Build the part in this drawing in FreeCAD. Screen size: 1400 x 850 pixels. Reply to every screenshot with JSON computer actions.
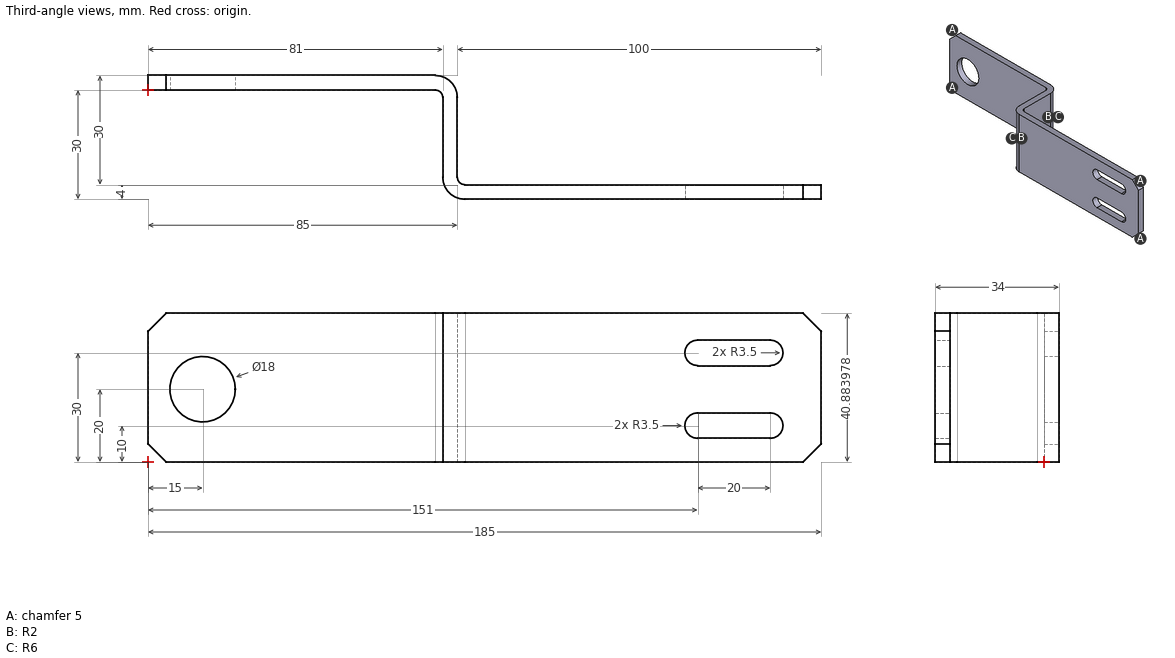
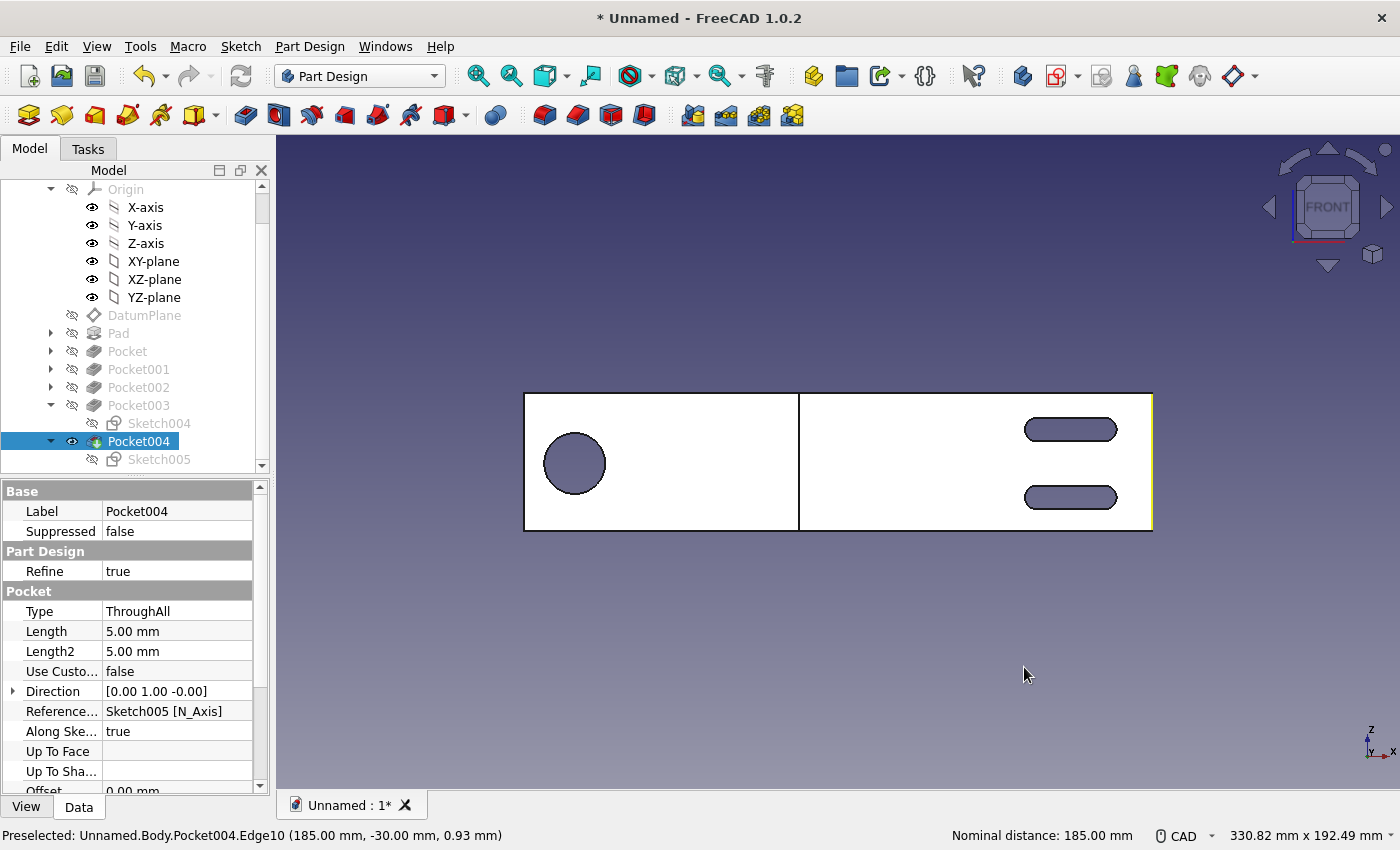
{"action": "scroll", "coordinate": [1152, 530], "scroll_direction": "up", "scroll_amount": 6}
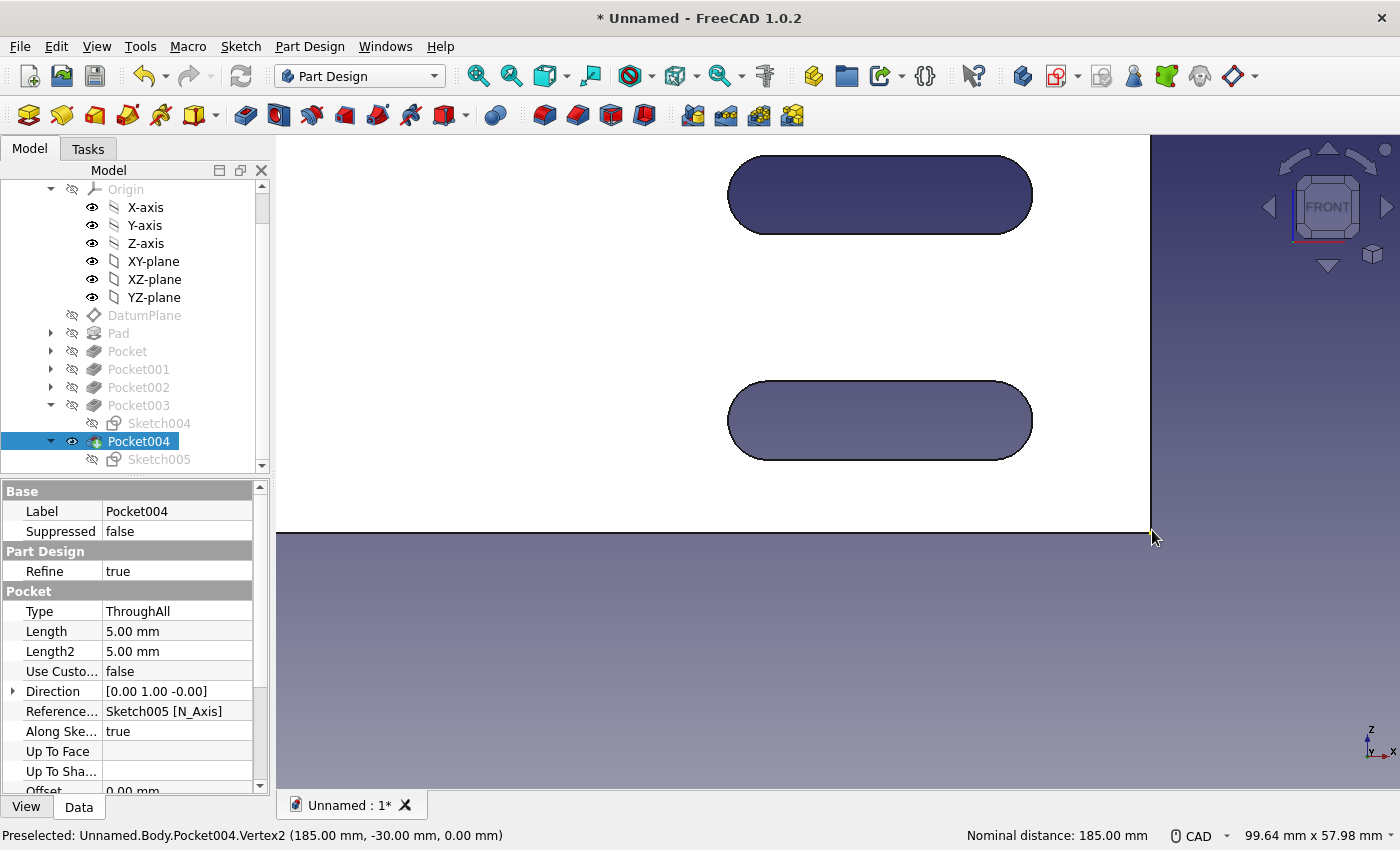
{"action": "key", "text": "v f"}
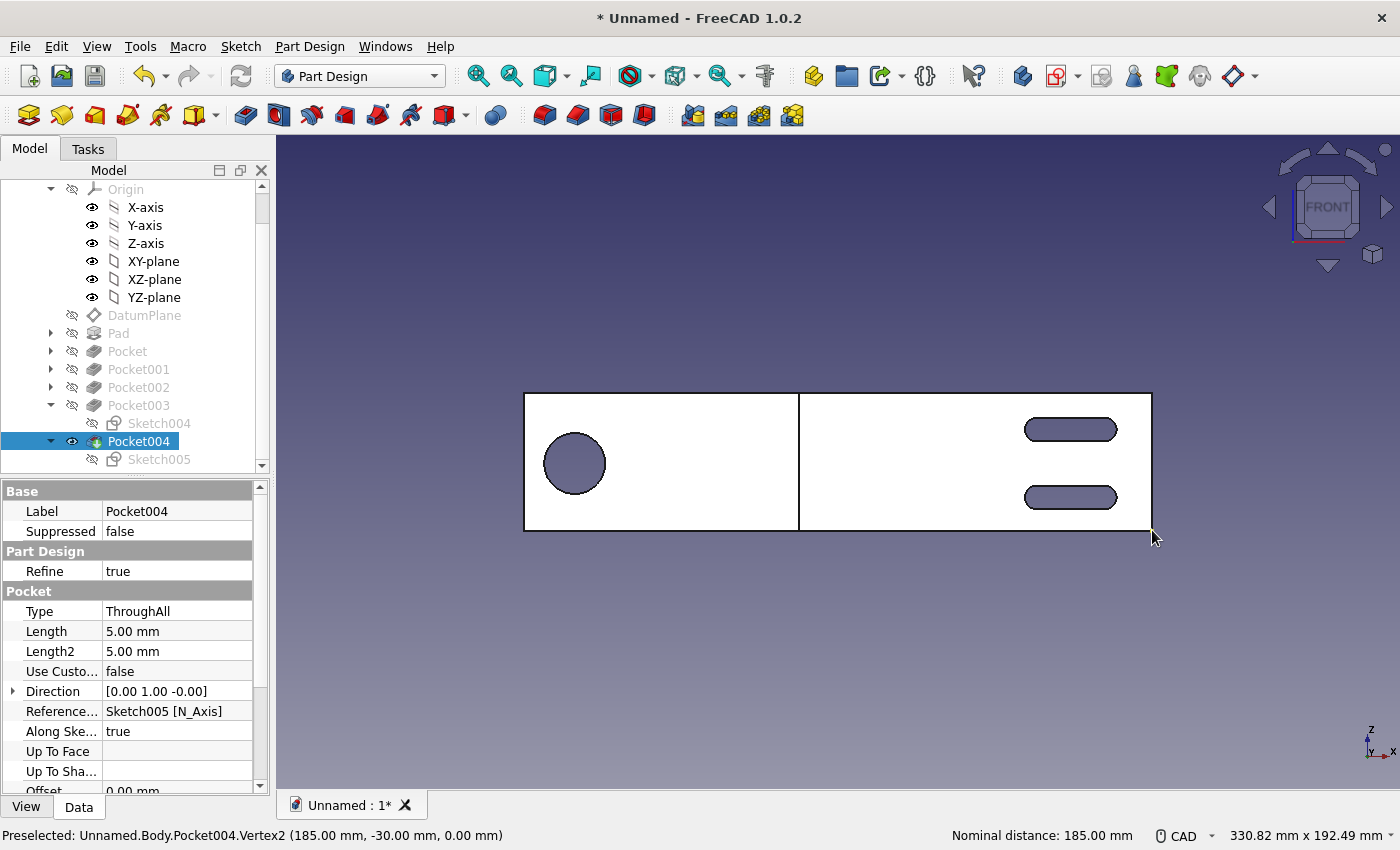
{"action": "key", "text": "3"}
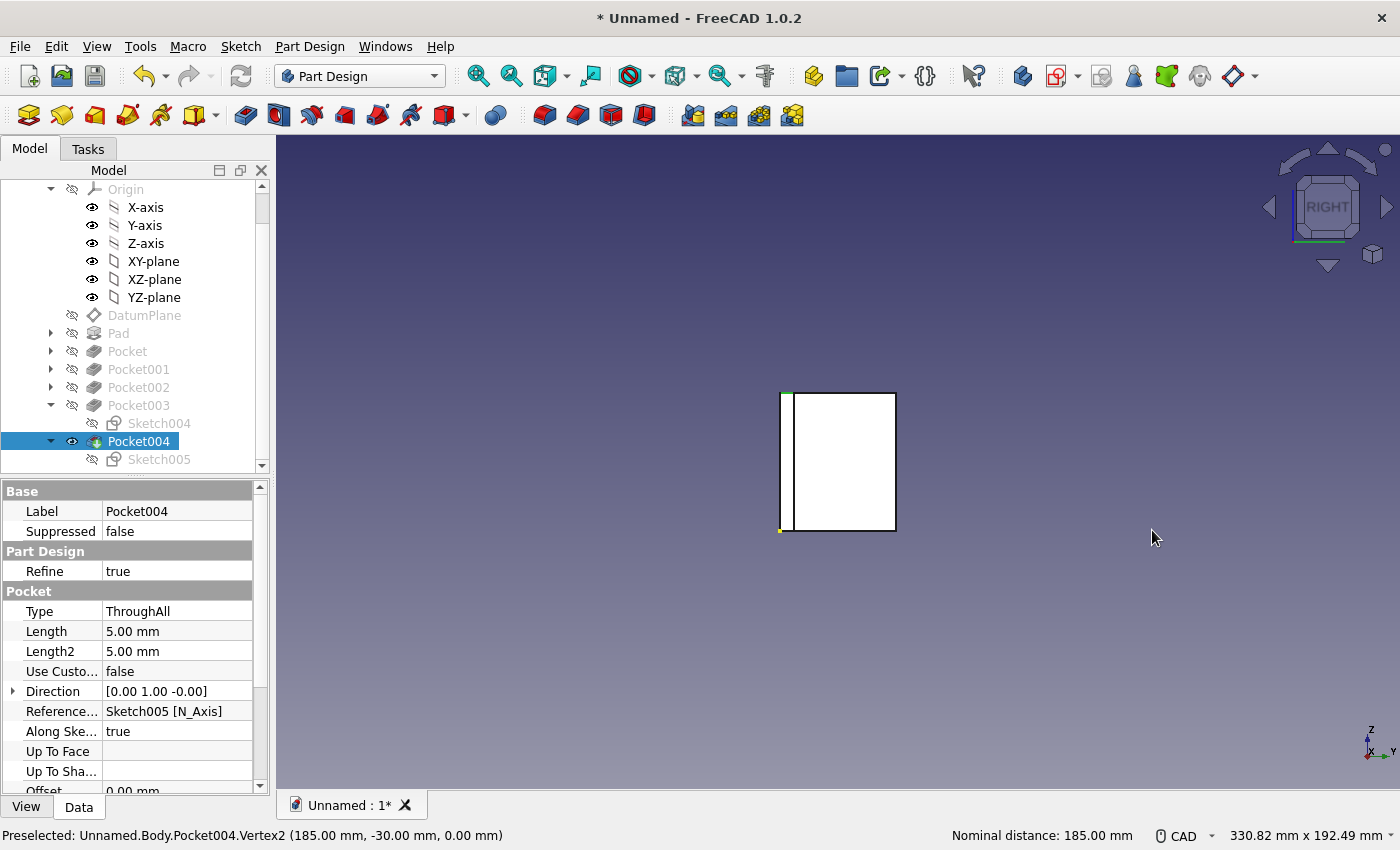
{"action": "left_click", "coordinate": [479, 76]}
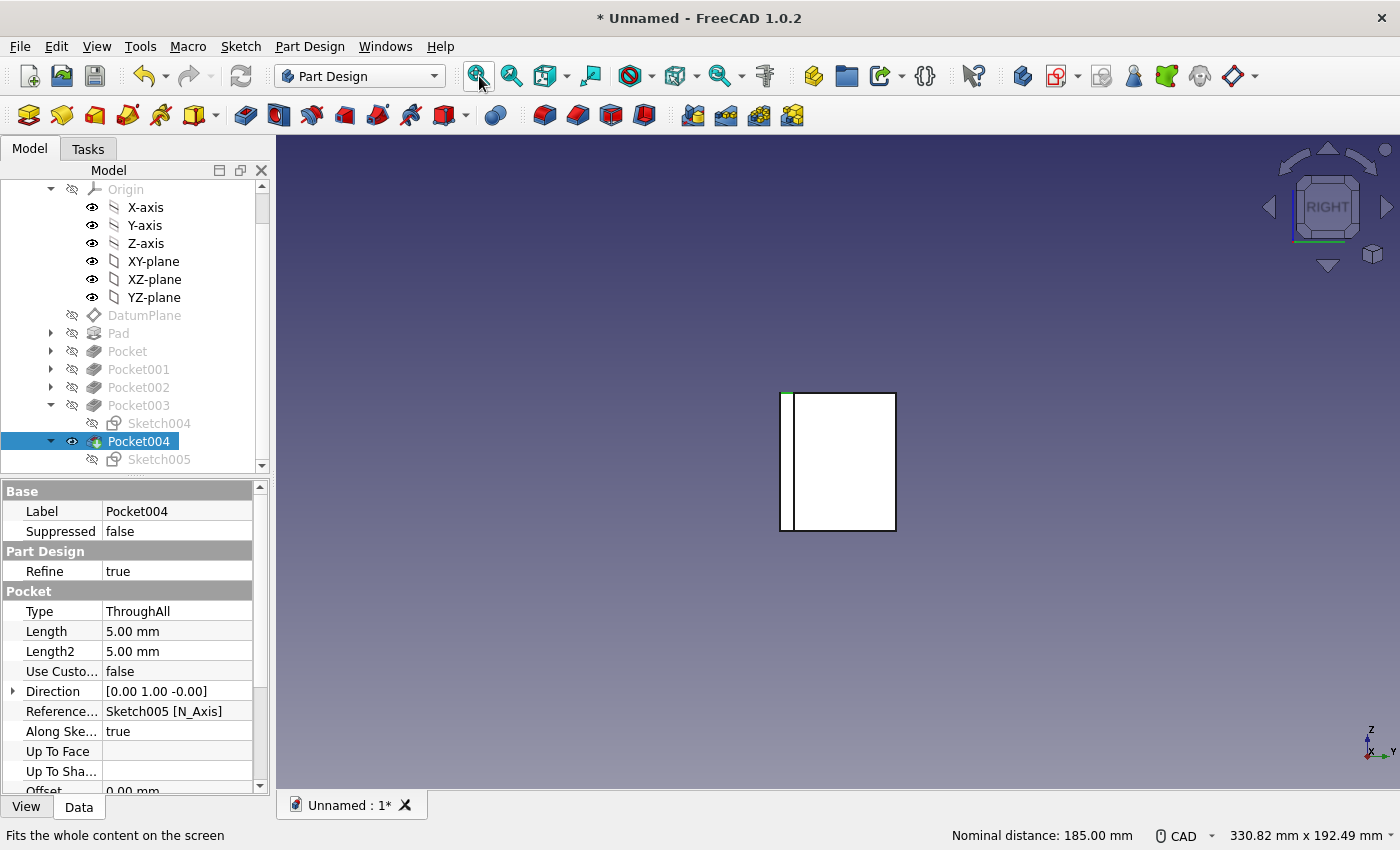
{"action": "left_click", "coordinate": [787, 530], "text": "ctrl"}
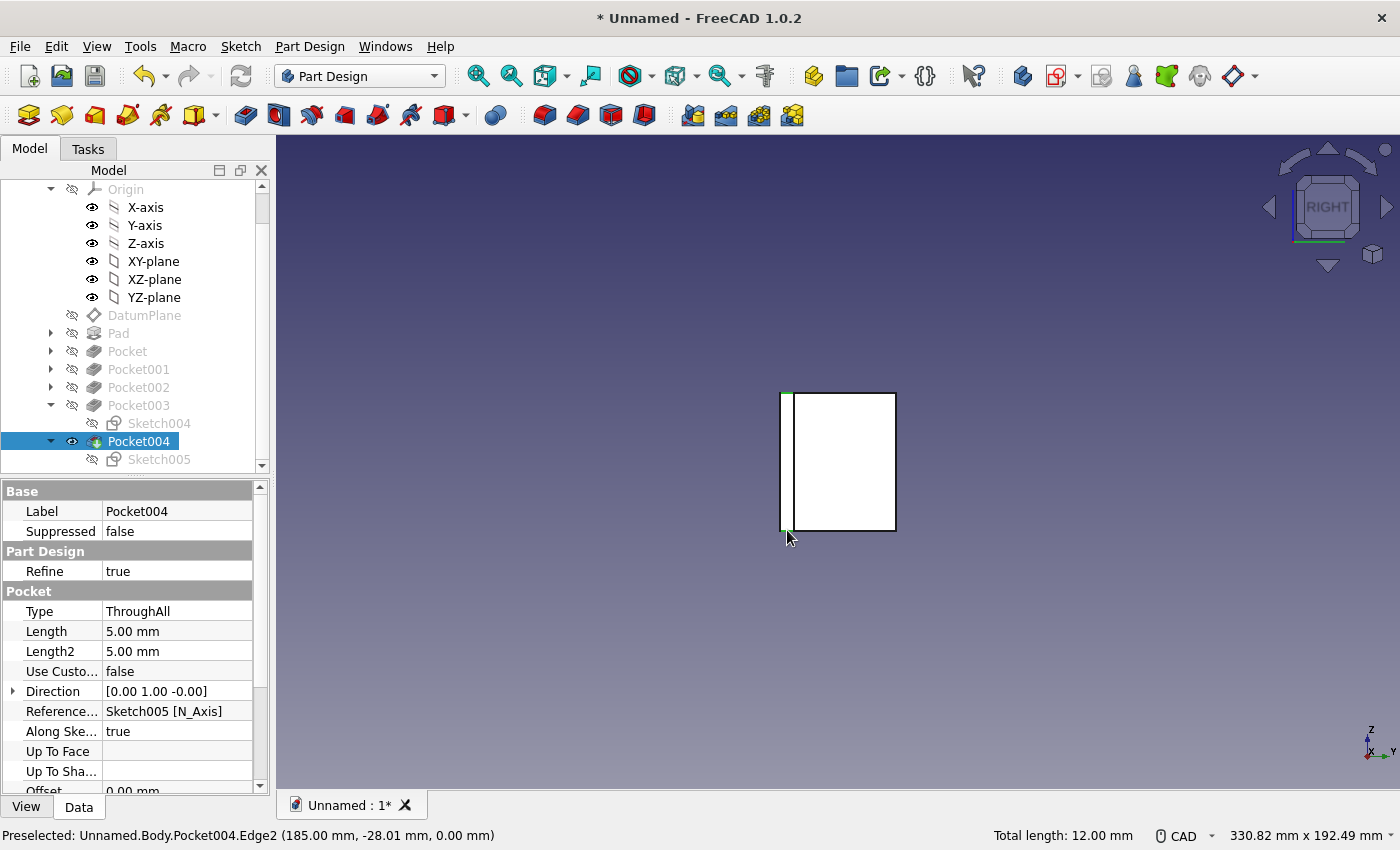
{"action": "scroll", "coordinate": [889, 530], "scroll_direction": "up", "scroll_amount": 6}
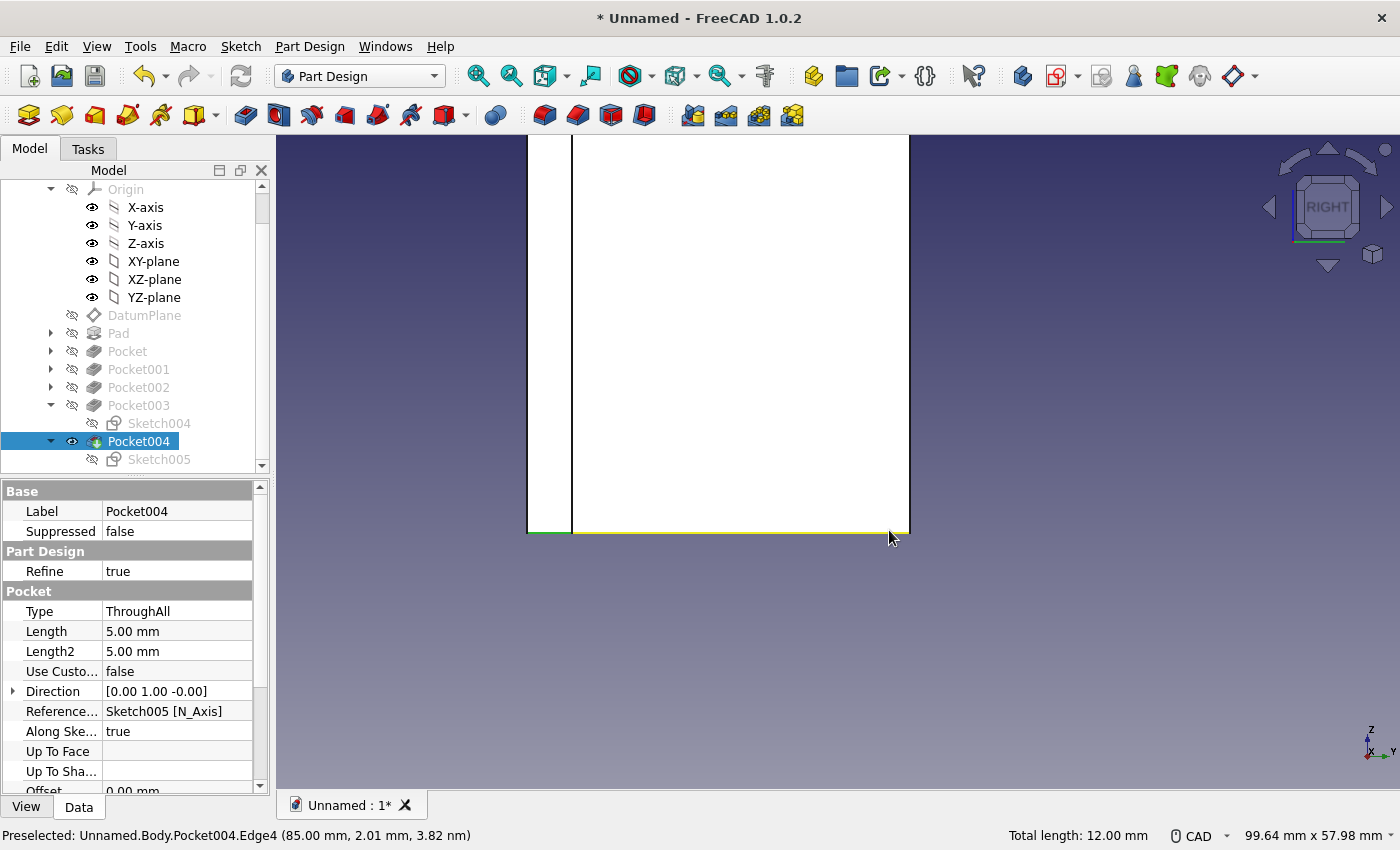
{"action": "key", "text": "v f"}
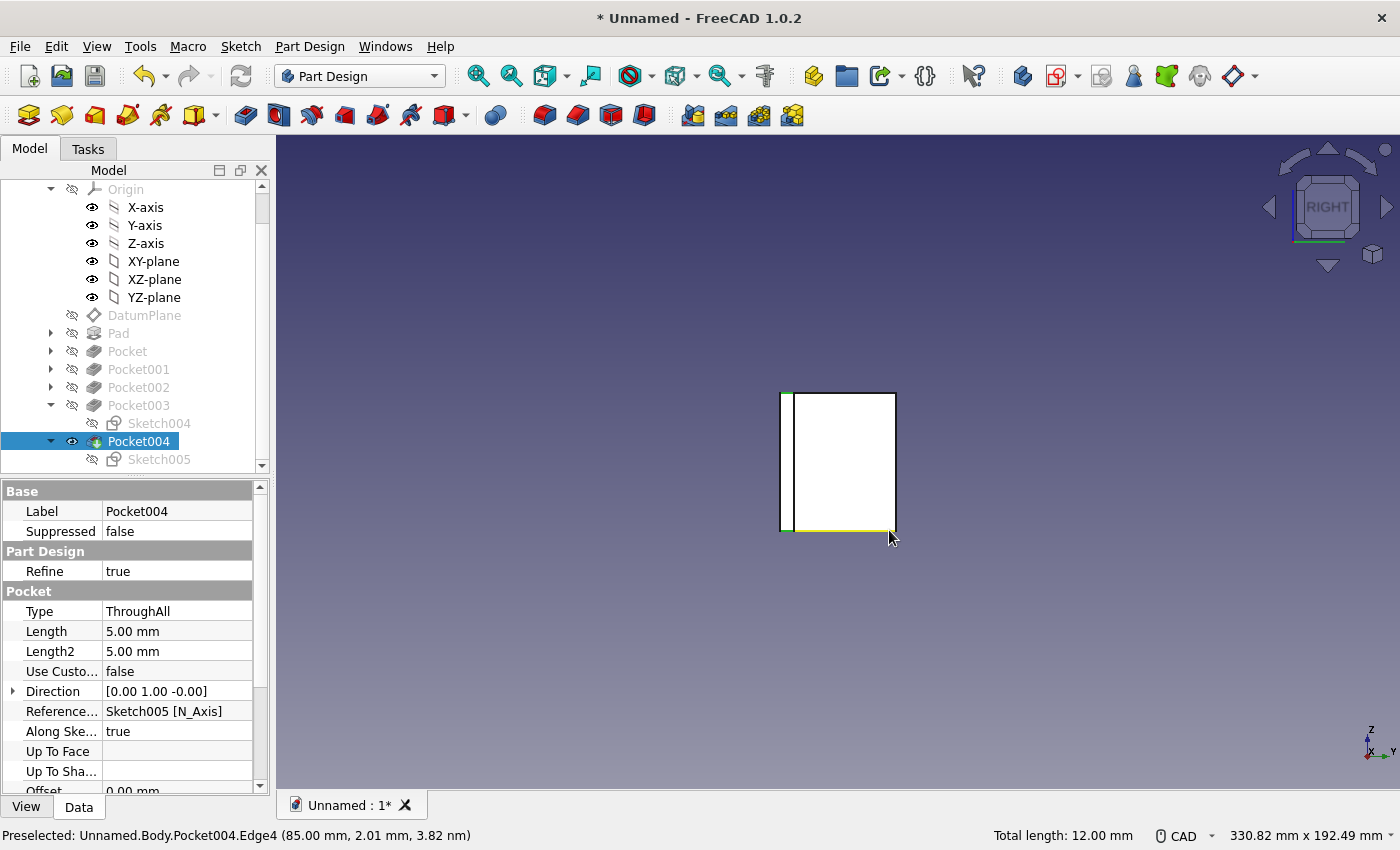
{"action": "key", "text": "5"}